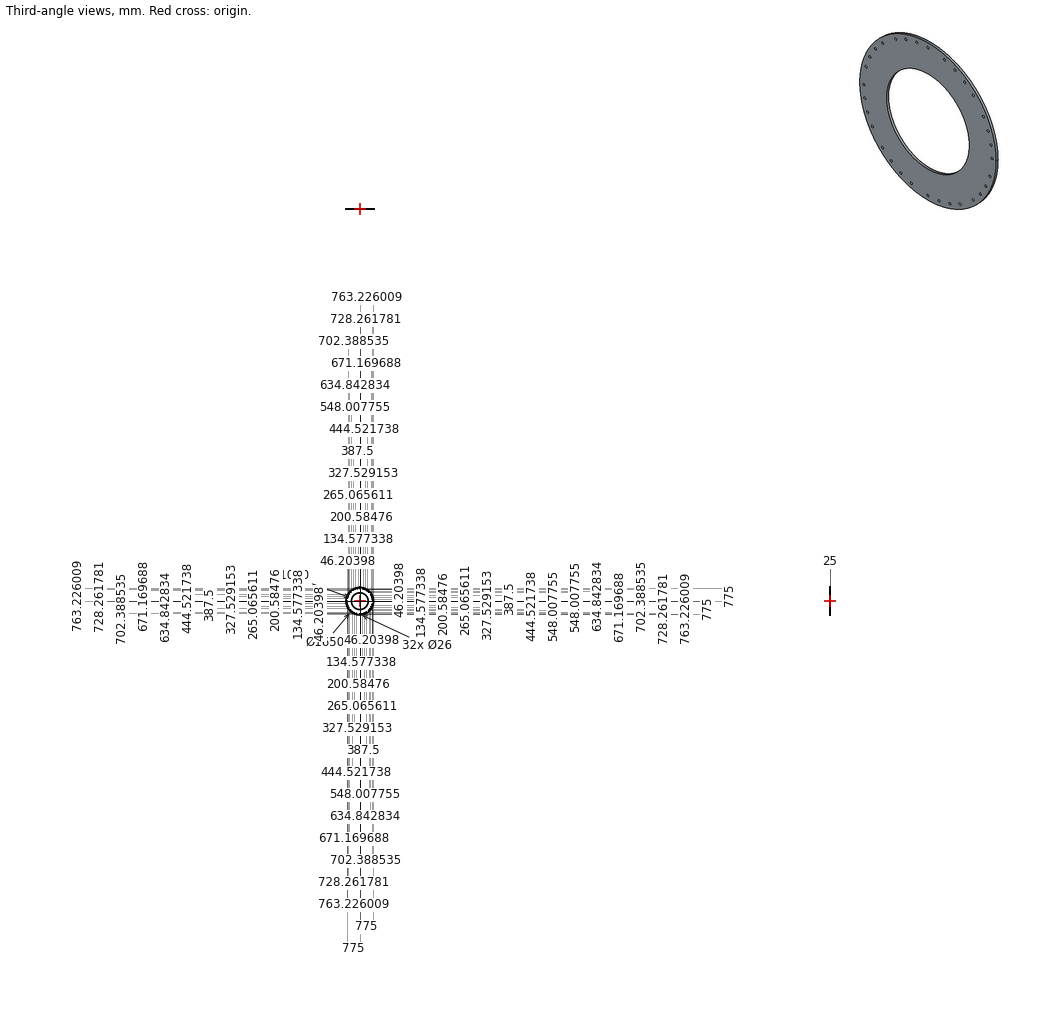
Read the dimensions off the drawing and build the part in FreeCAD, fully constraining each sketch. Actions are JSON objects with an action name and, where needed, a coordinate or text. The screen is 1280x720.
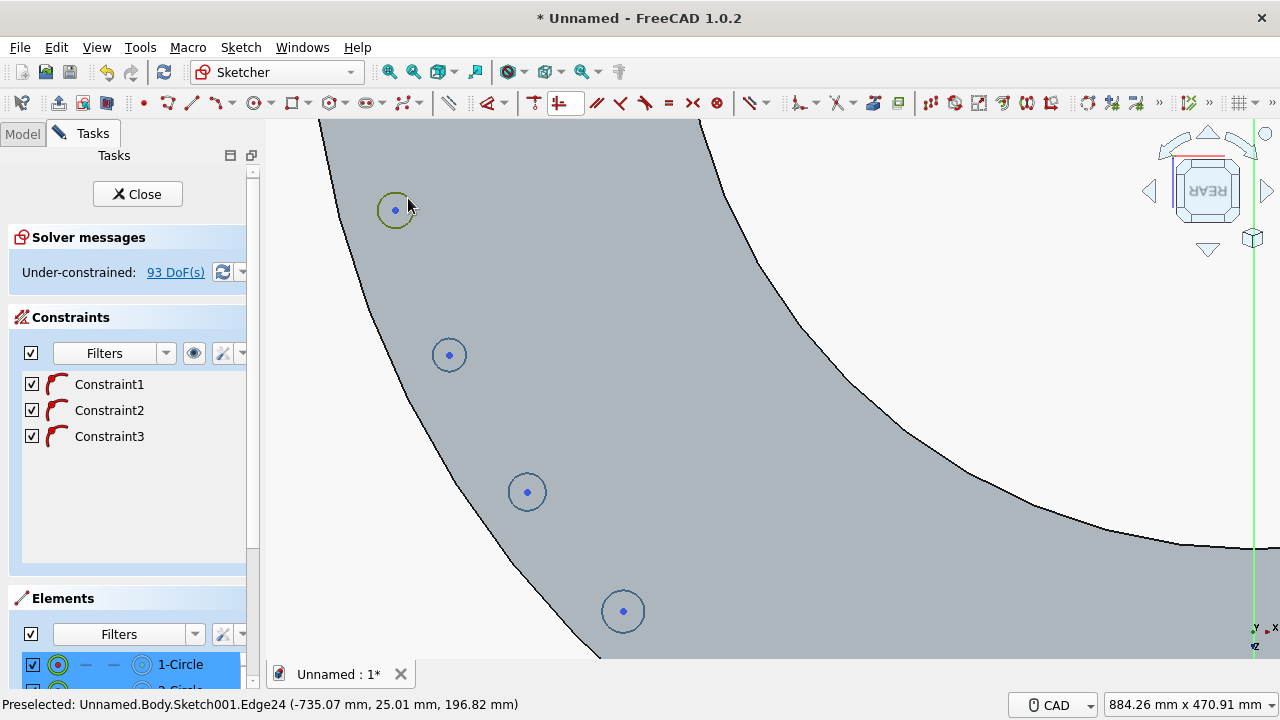
{"action": "scroll", "coordinate": [565, 493], "scroll_direction": "down", "scroll_amount": 8}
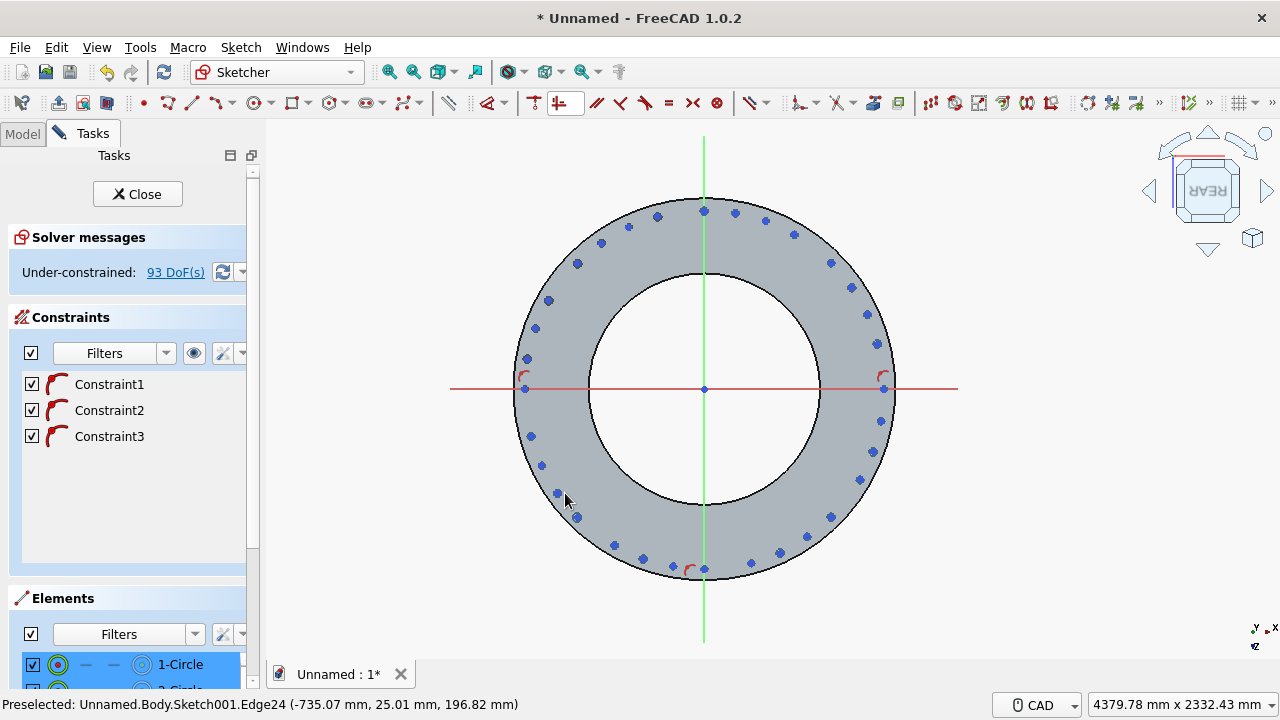
{"action": "scroll", "coordinate": [527, 387], "scroll_direction": "up", "scroll_amount": 9}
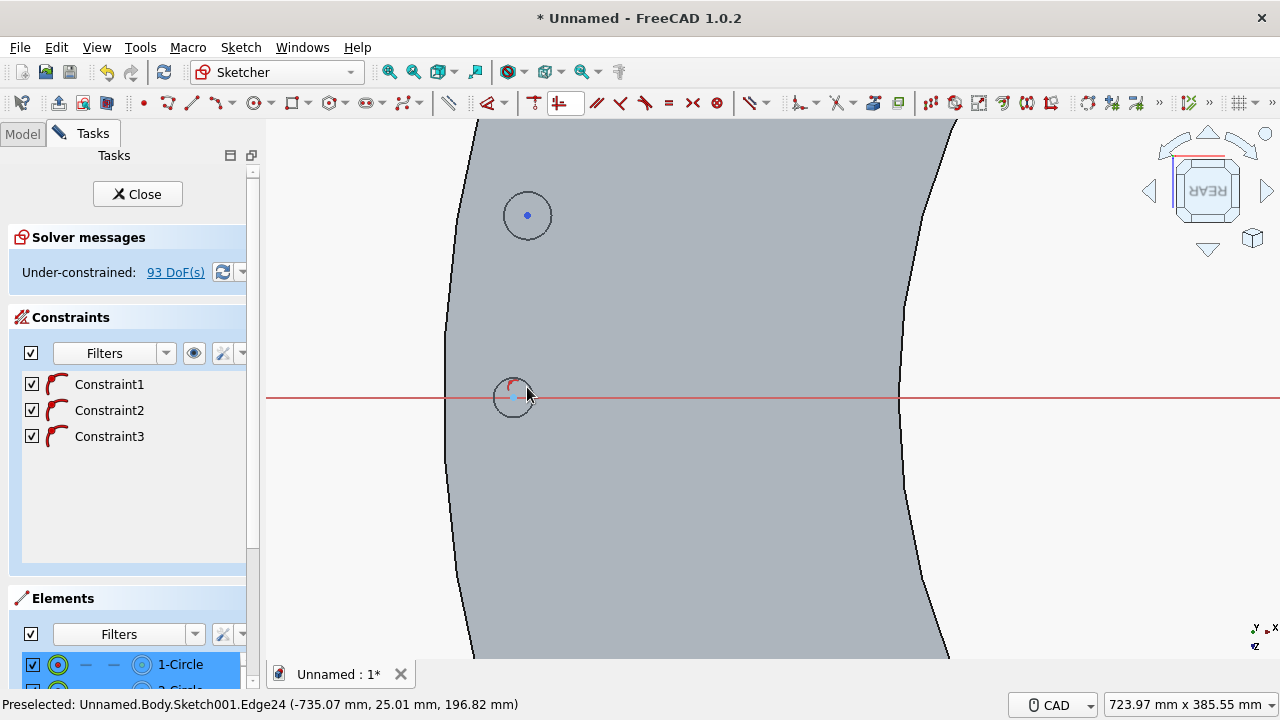
{"action": "left_click", "coordinate": [527, 384]}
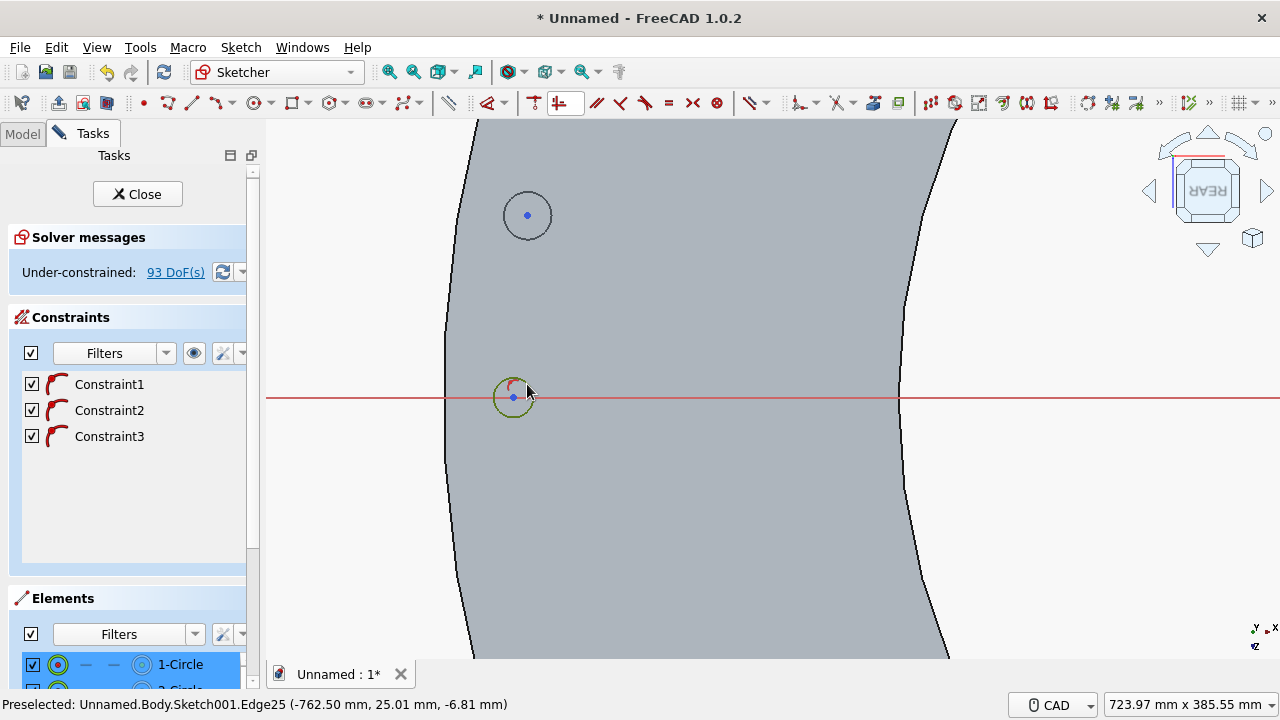
{"action": "left_click", "coordinate": [545, 199]}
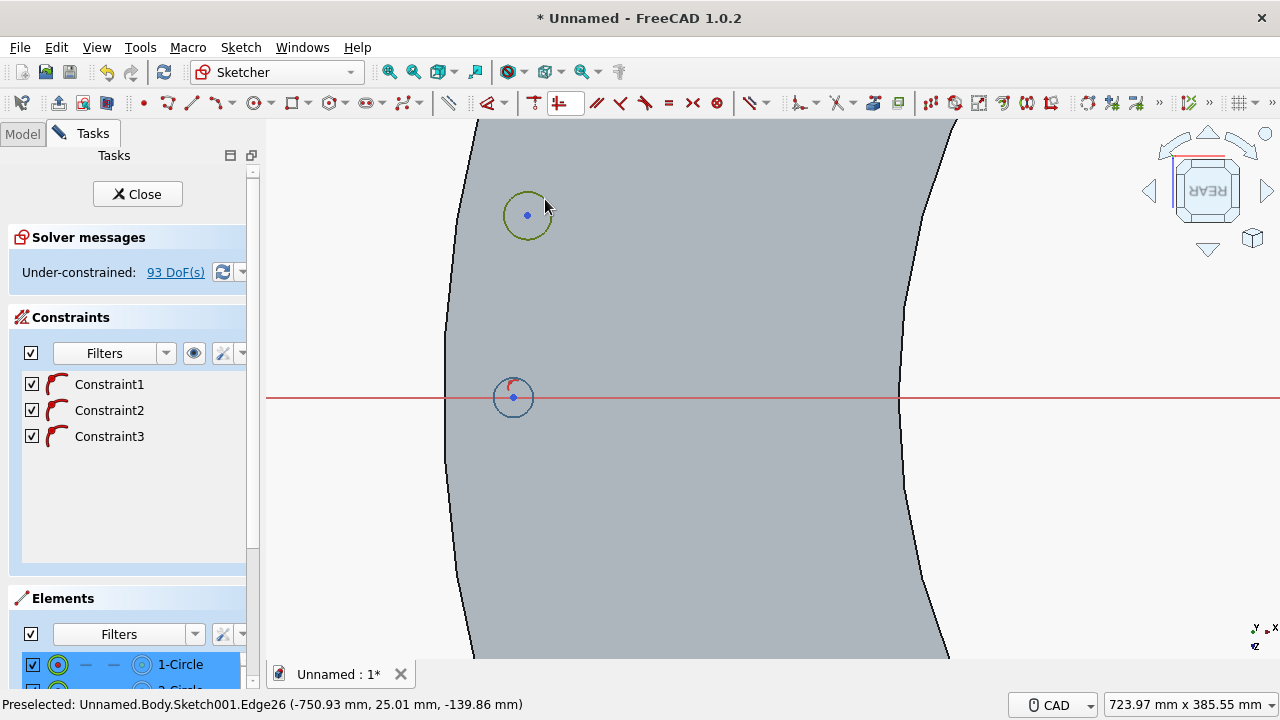
{"action": "scroll", "coordinate": [527, 387], "scroll_direction": "down", "scroll_amount": 9}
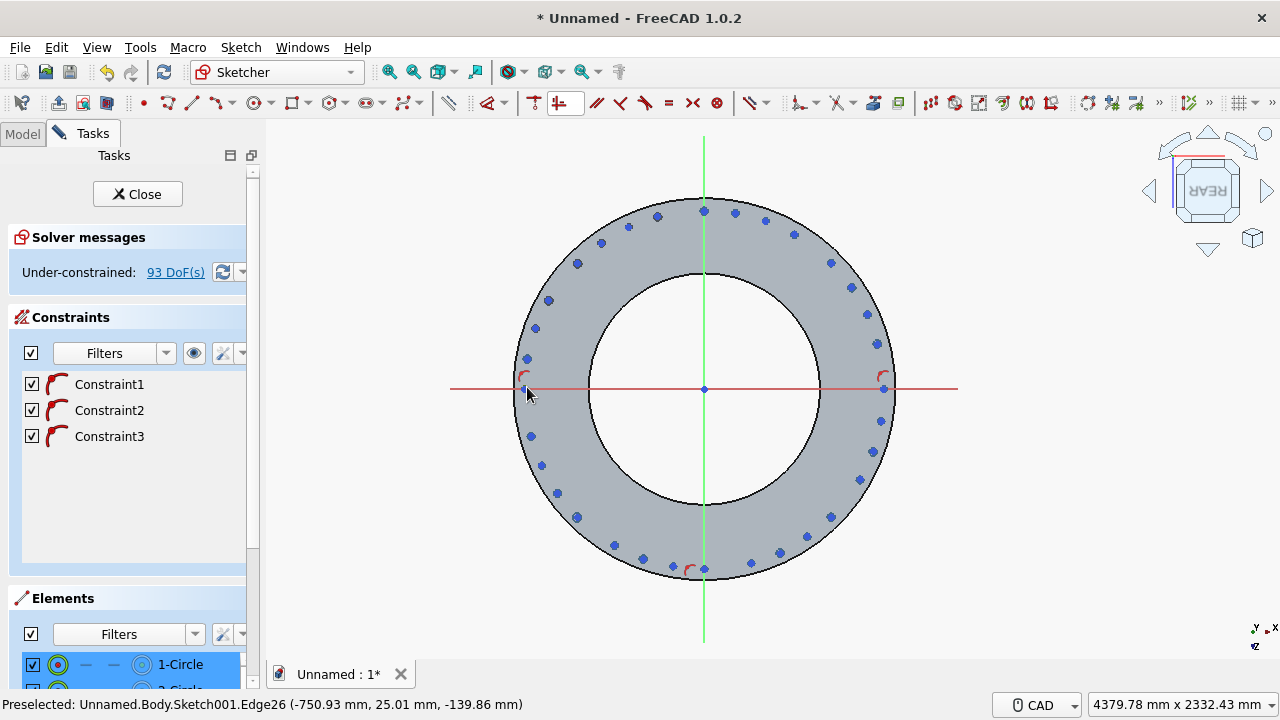
{"action": "scroll", "coordinate": [538, 326], "scroll_direction": "up", "scroll_amount": 7}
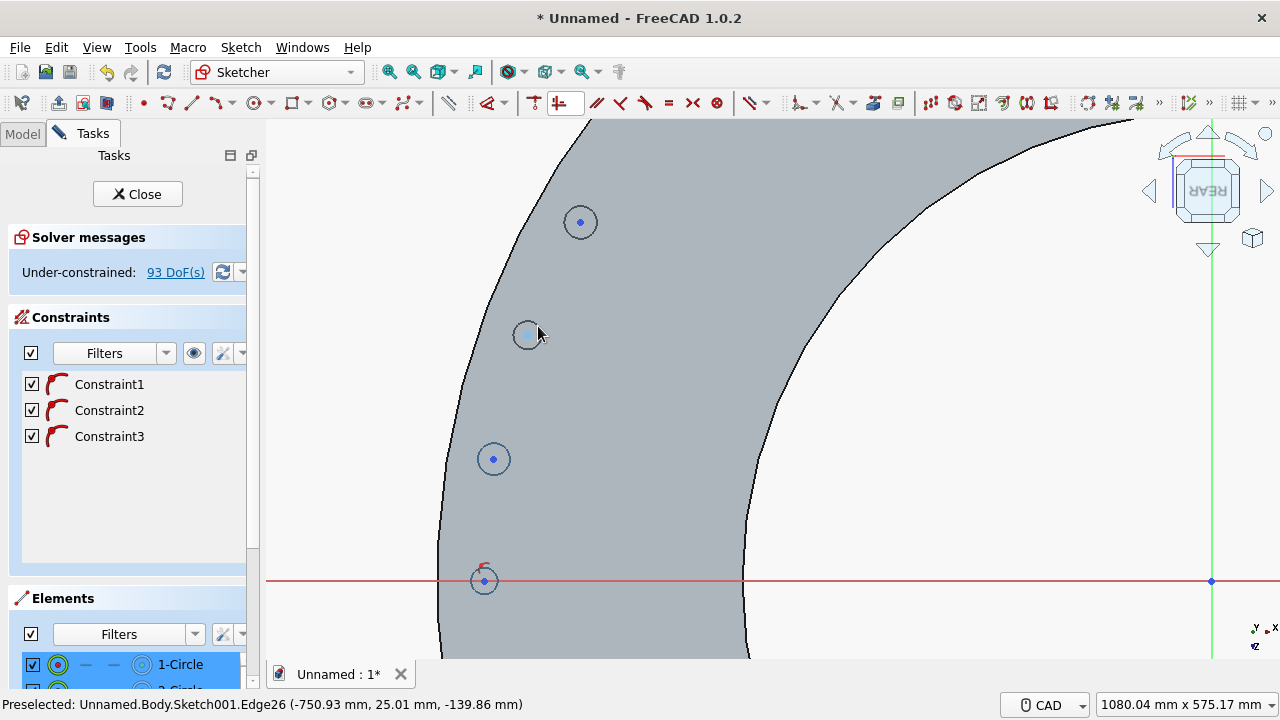
{"action": "left_click", "coordinate": [538, 325]}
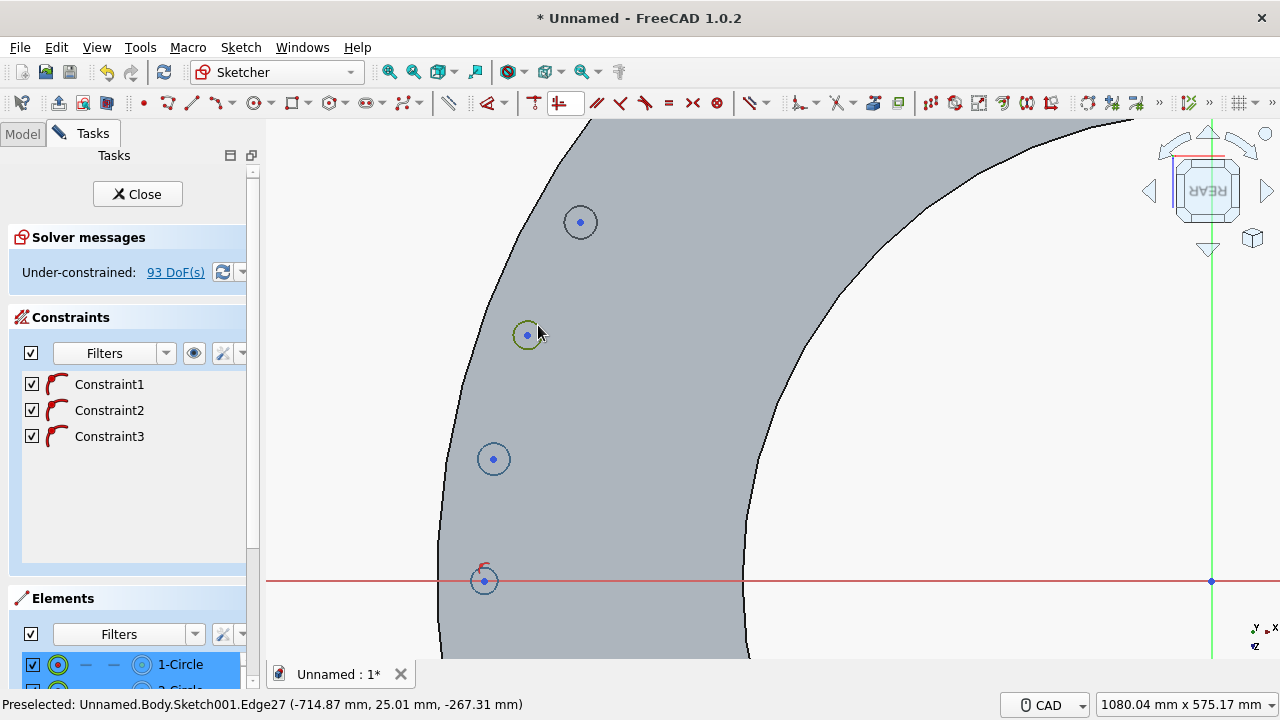
{"action": "left_click", "coordinate": [592, 211]}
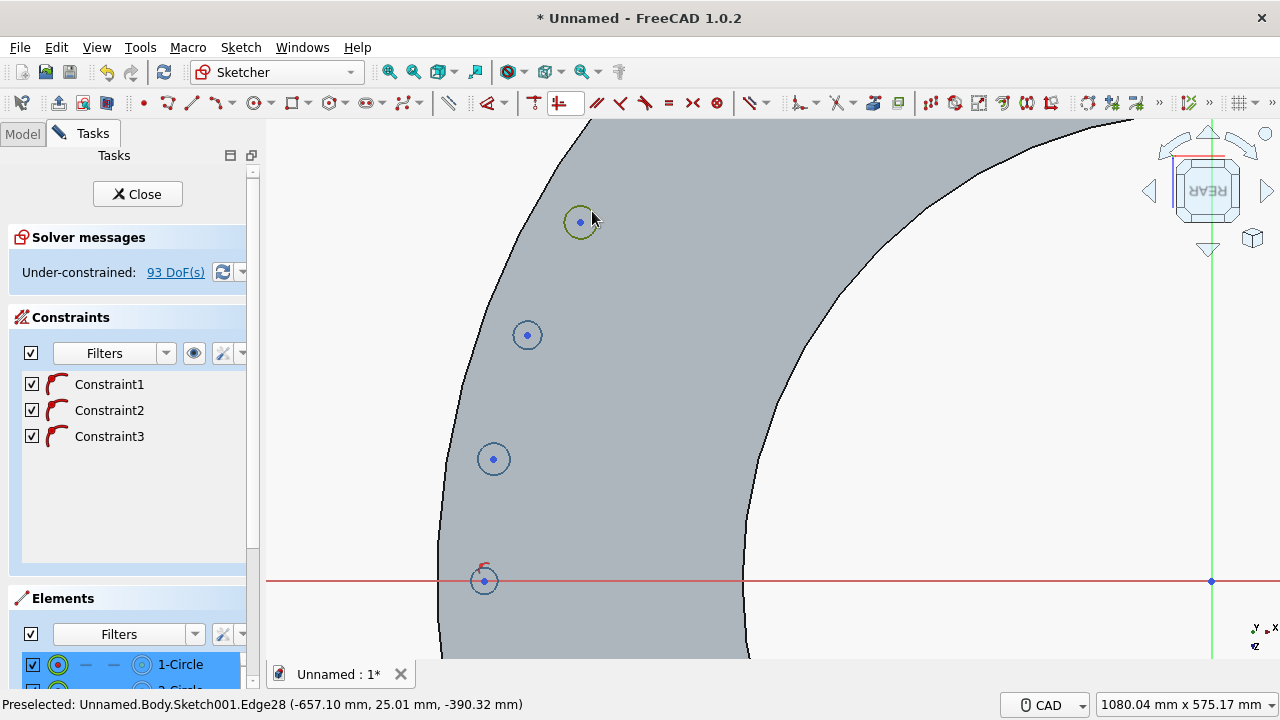
{"action": "scroll", "coordinate": [538, 326], "scroll_direction": "down", "scroll_amount": 7}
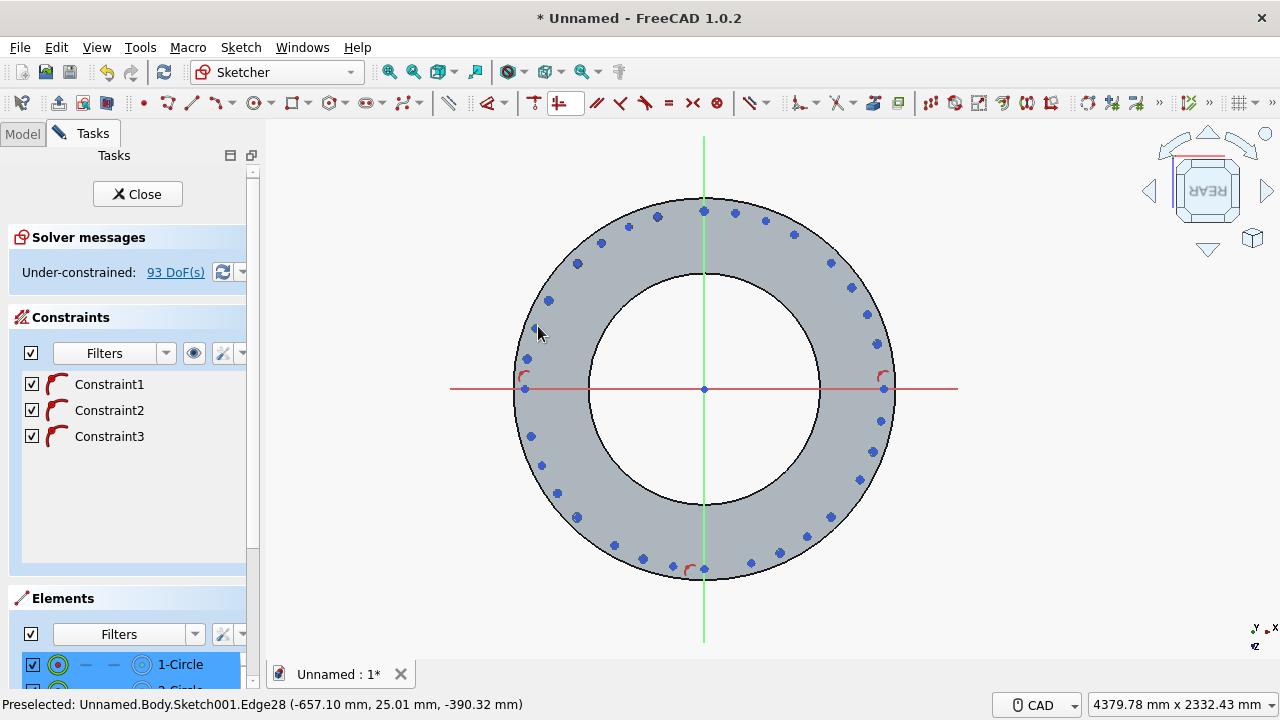
{"action": "scroll", "coordinate": [581, 261], "scroll_direction": "up", "scroll_amount": 7}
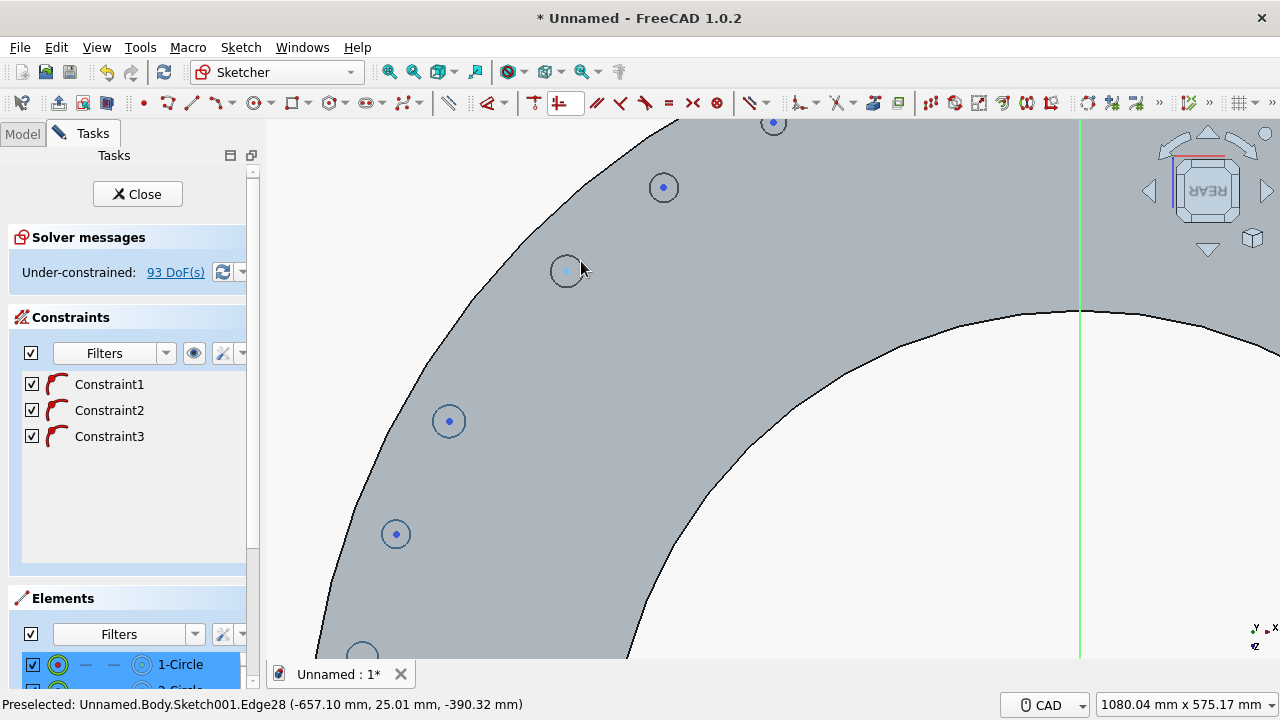
{"action": "left_click", "coordinate": [578, 260]}